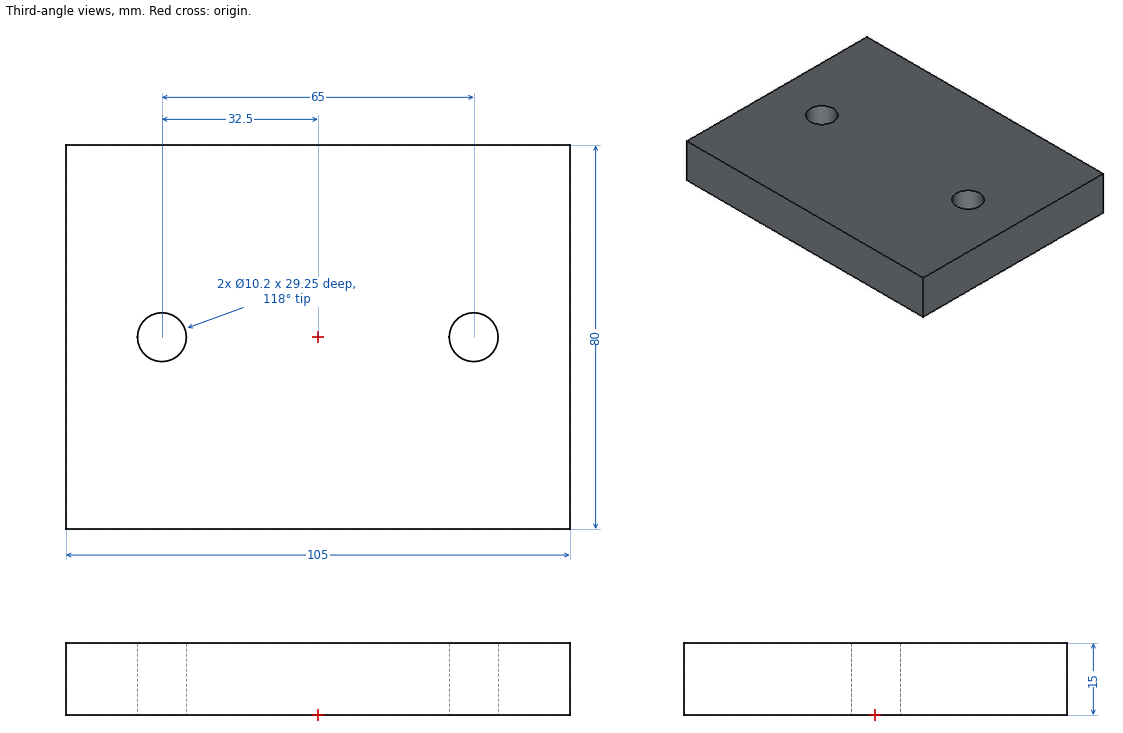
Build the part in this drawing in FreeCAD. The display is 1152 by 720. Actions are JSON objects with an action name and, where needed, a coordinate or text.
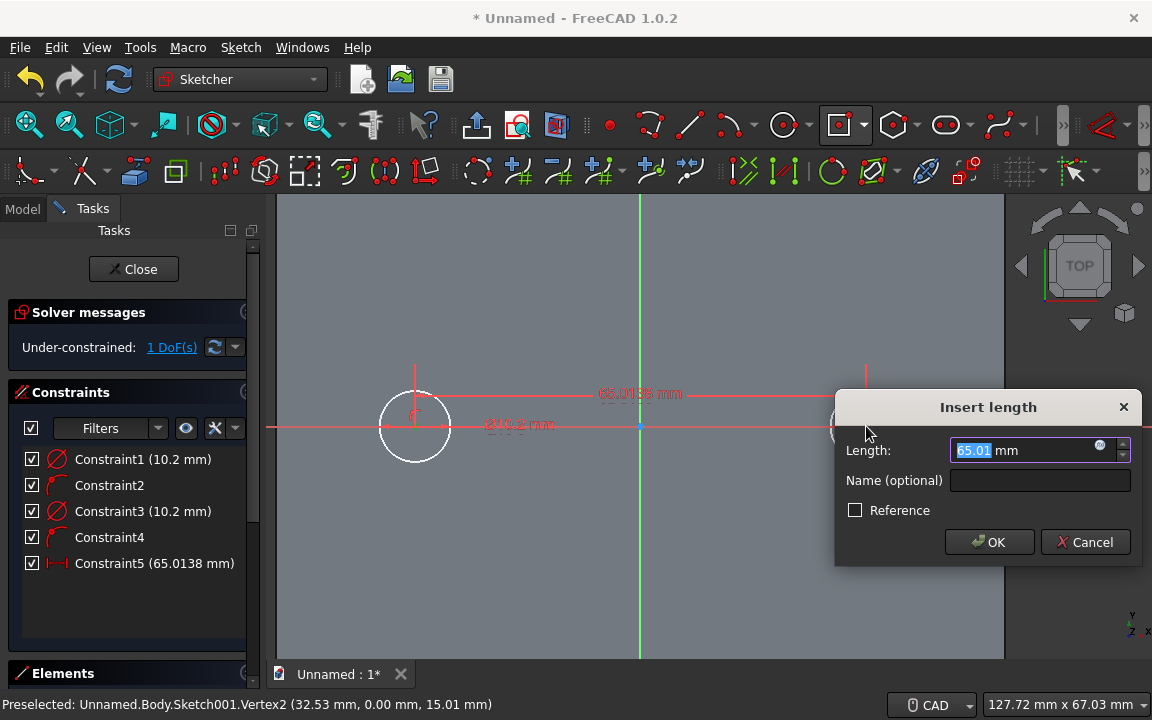
{"action": "type", "text": "65"}
{"action": "key", "text": "Return"}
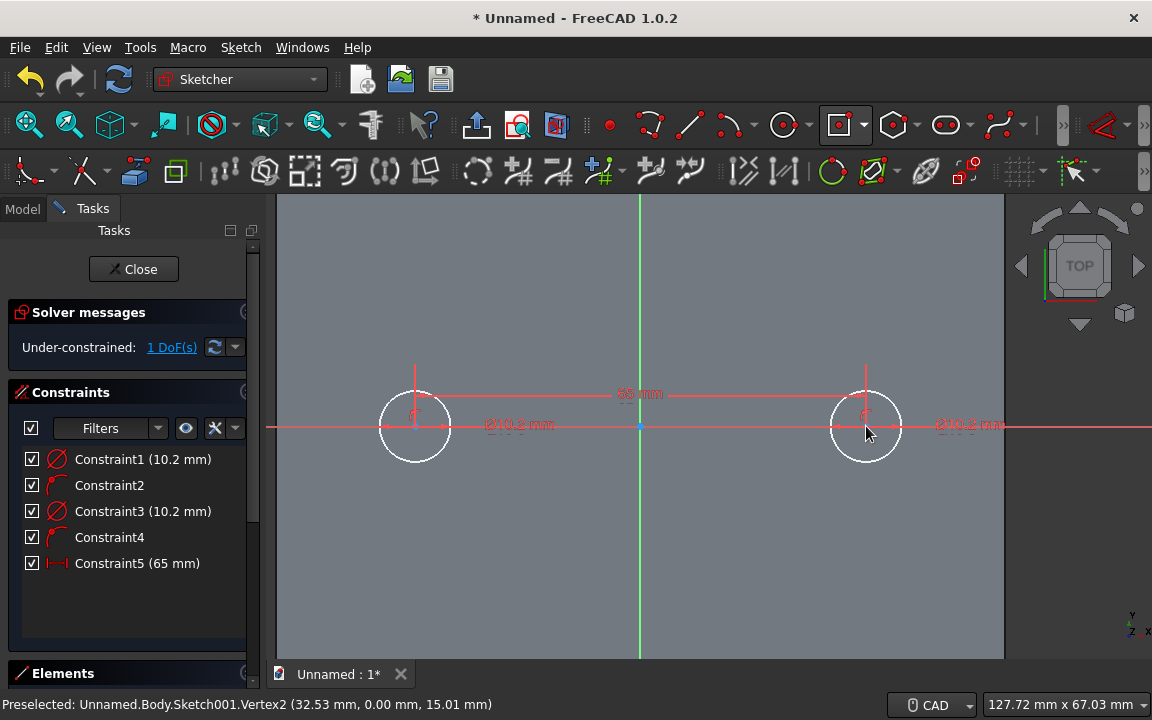
{"action": "left_click", "coordinate": [415, 426]}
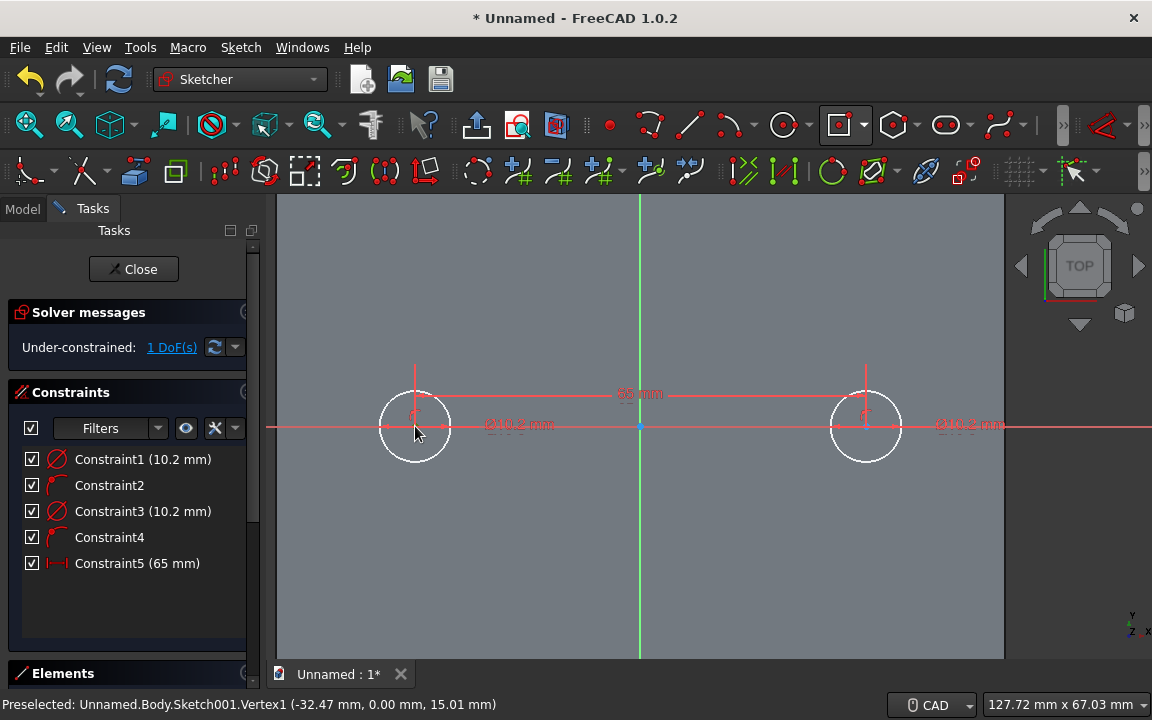
{"action": "left_click", "coordinate": [1130, 126]}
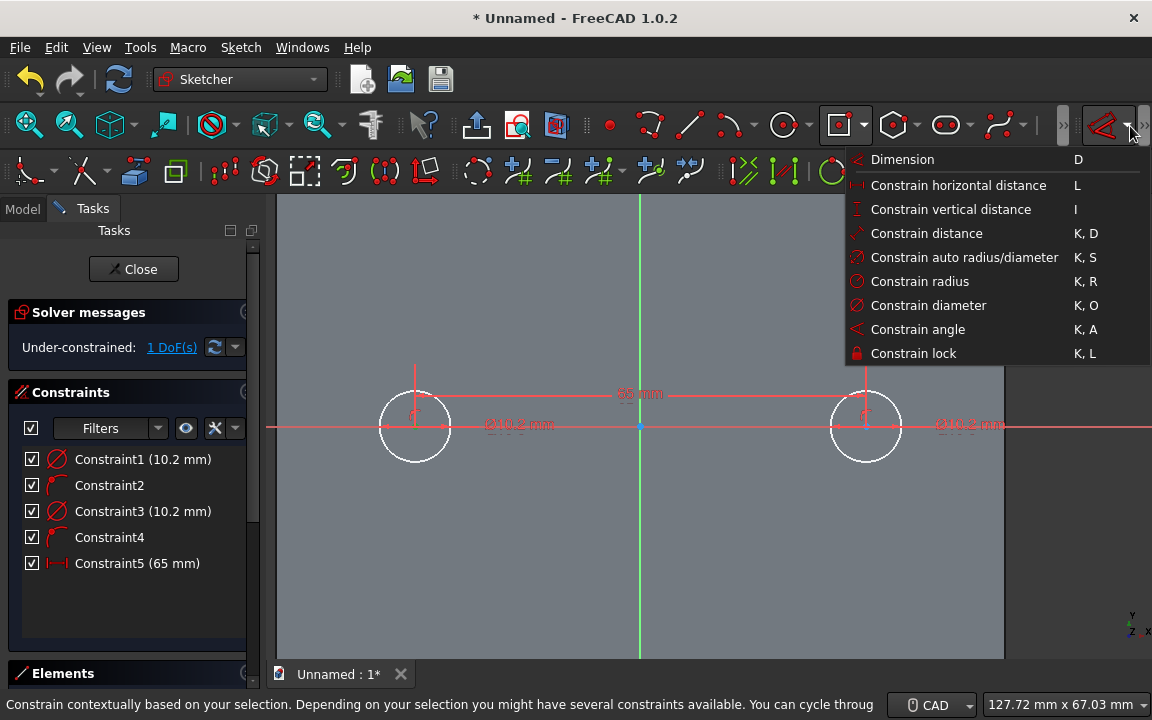
{"action": "left_click", "coordinate": [998, 185]}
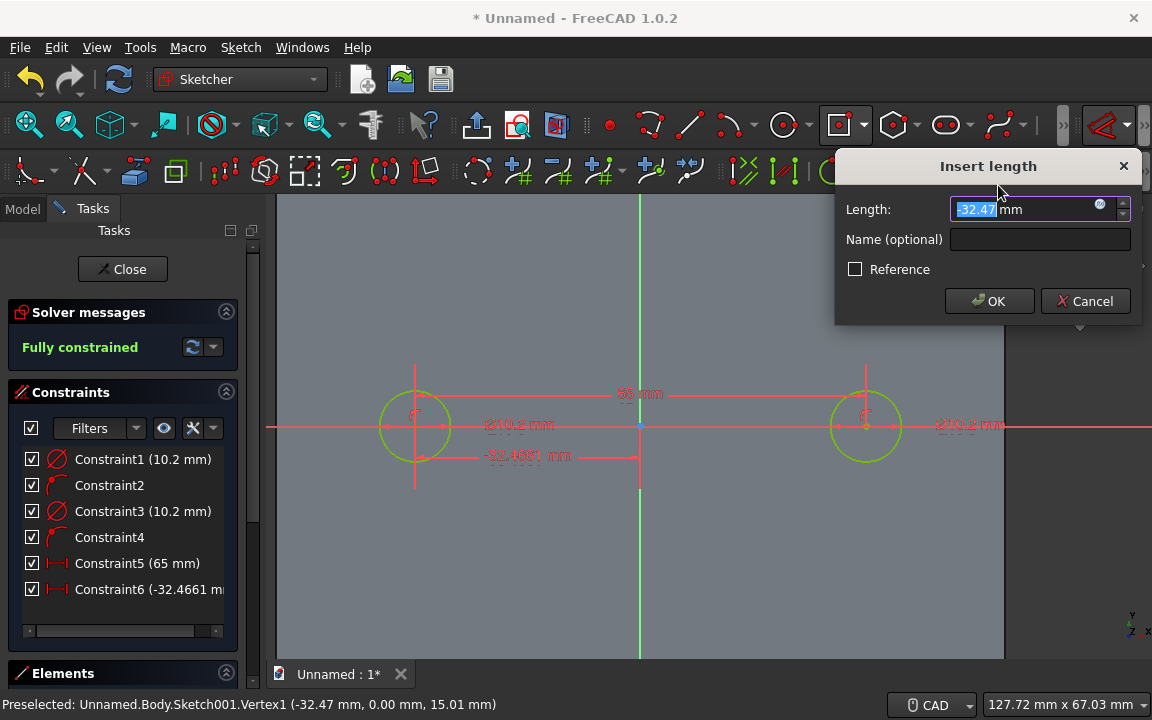
{"action": "type", "text": "-32.5"}
{"action": "key", "text": "Return"}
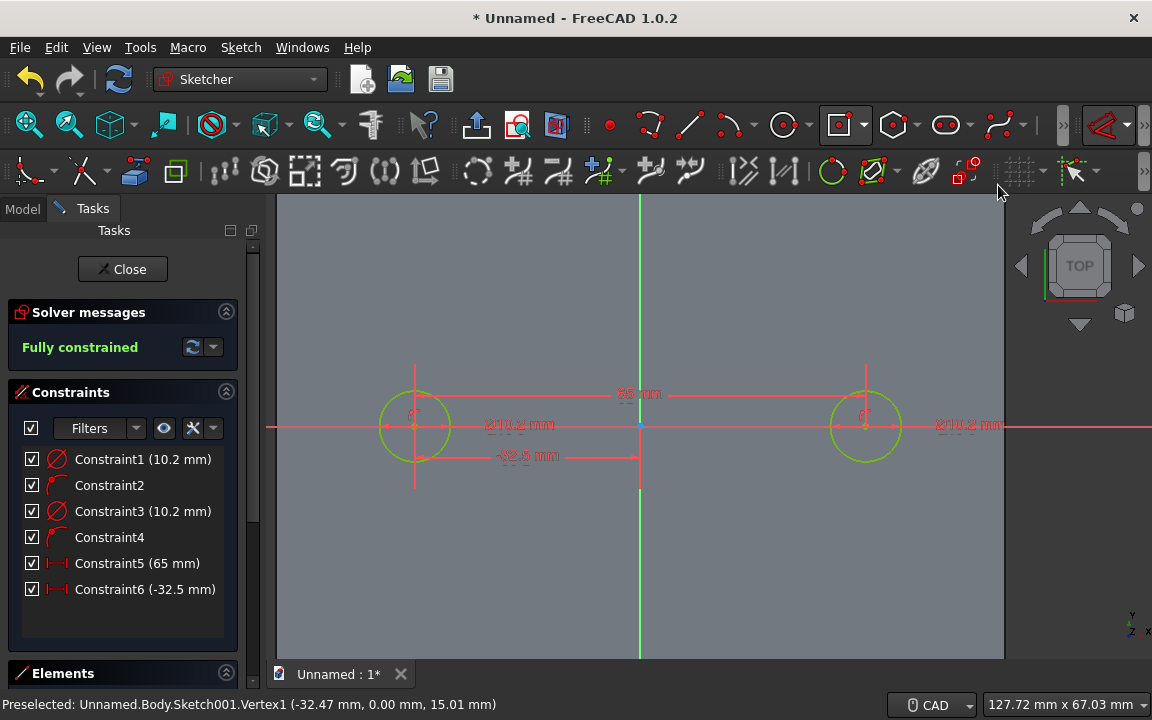
{"action": "left_click", "coordinate": [123, 269]}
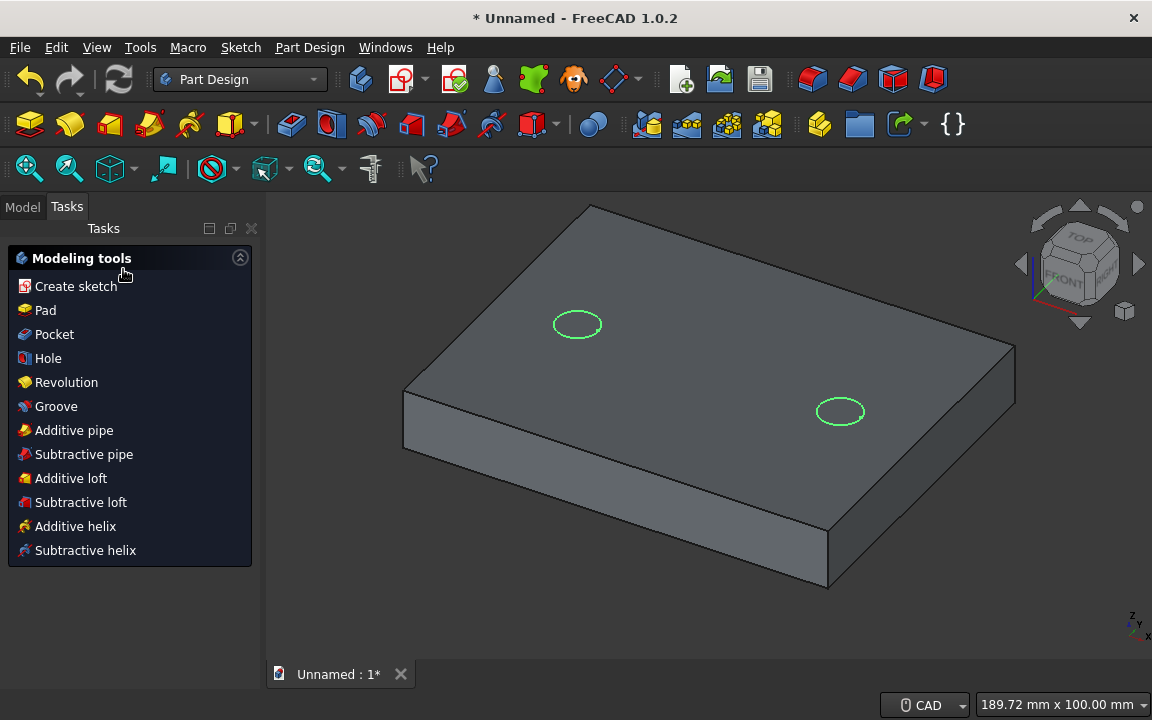
{"action": "left_click", "coordinate": [332, 124]}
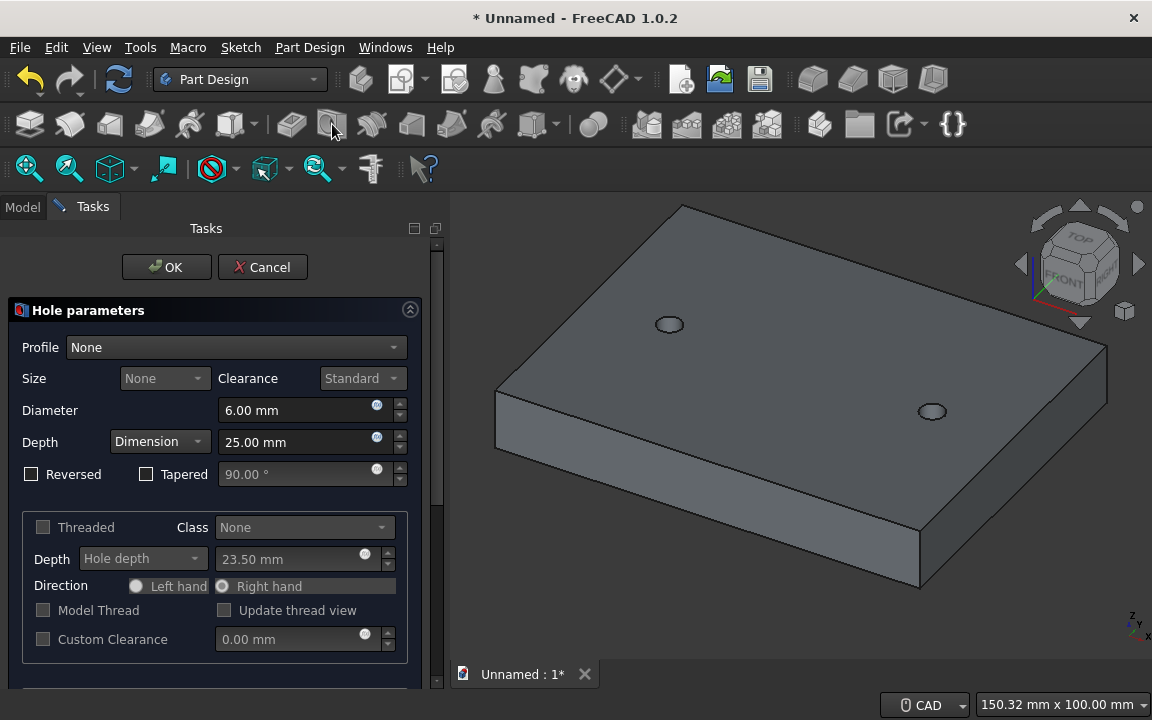
{"action": "triple_click", "coordinate": [305, 410]}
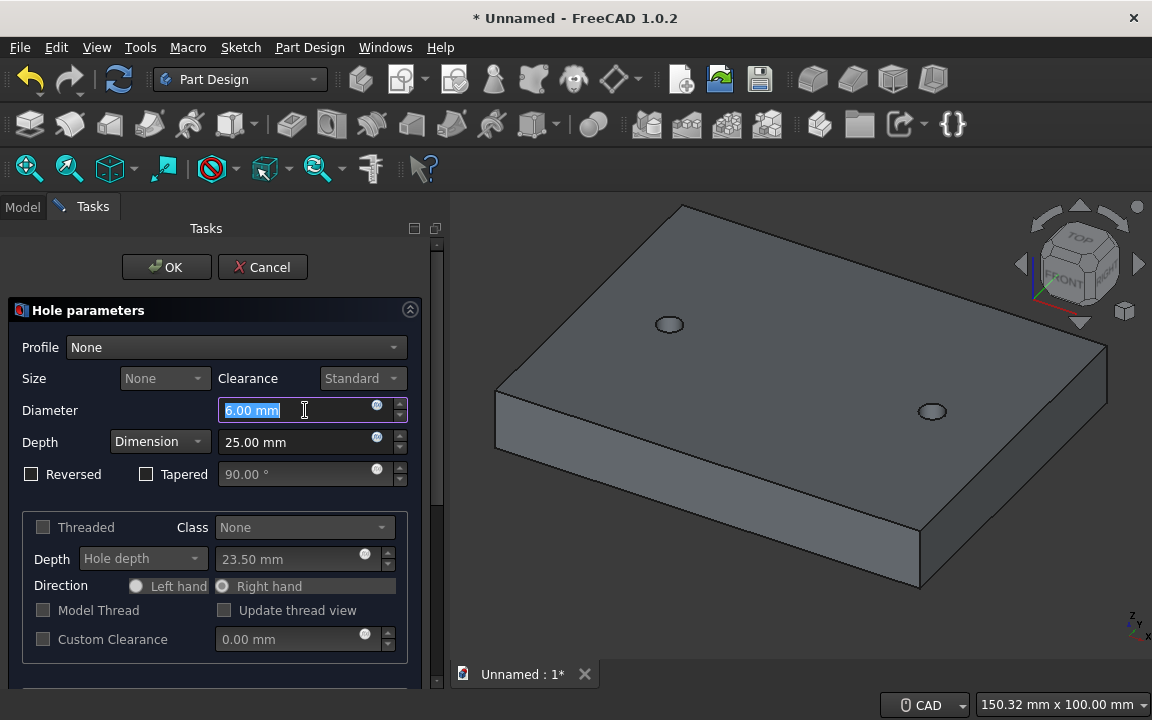
{"action": "type", "text": "10.2"}
{"action": "key", "text": "Tab"}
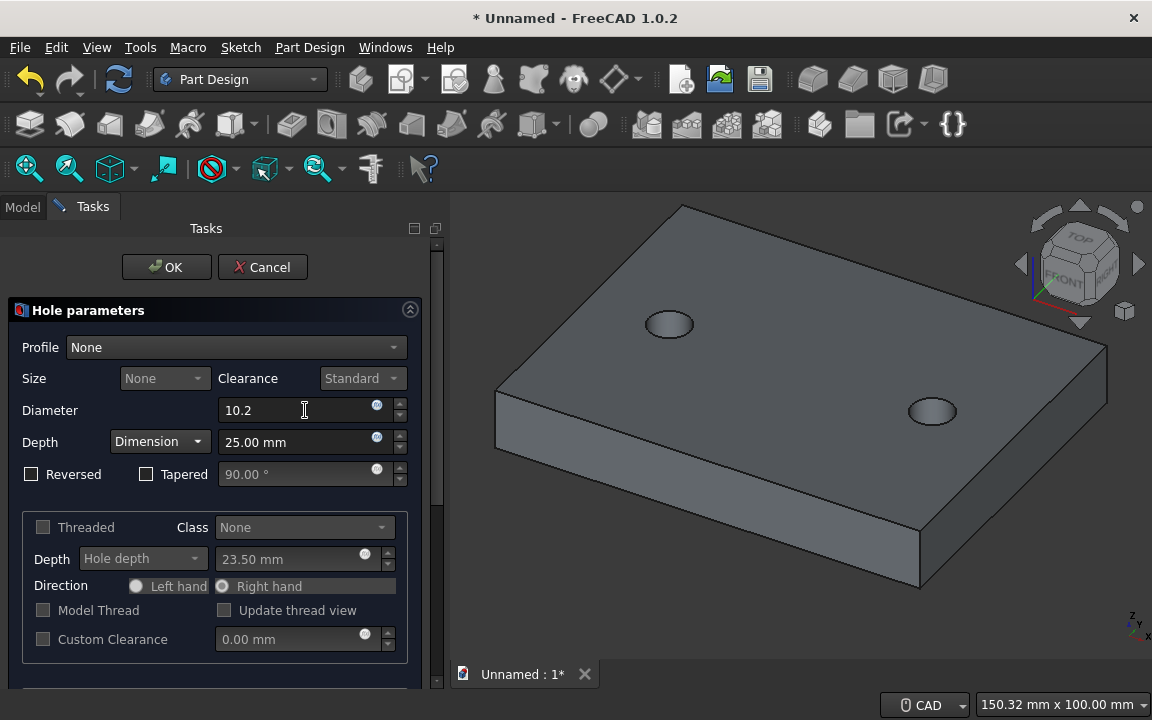
{"action": "triple_click", "coordinate": [305, 442]}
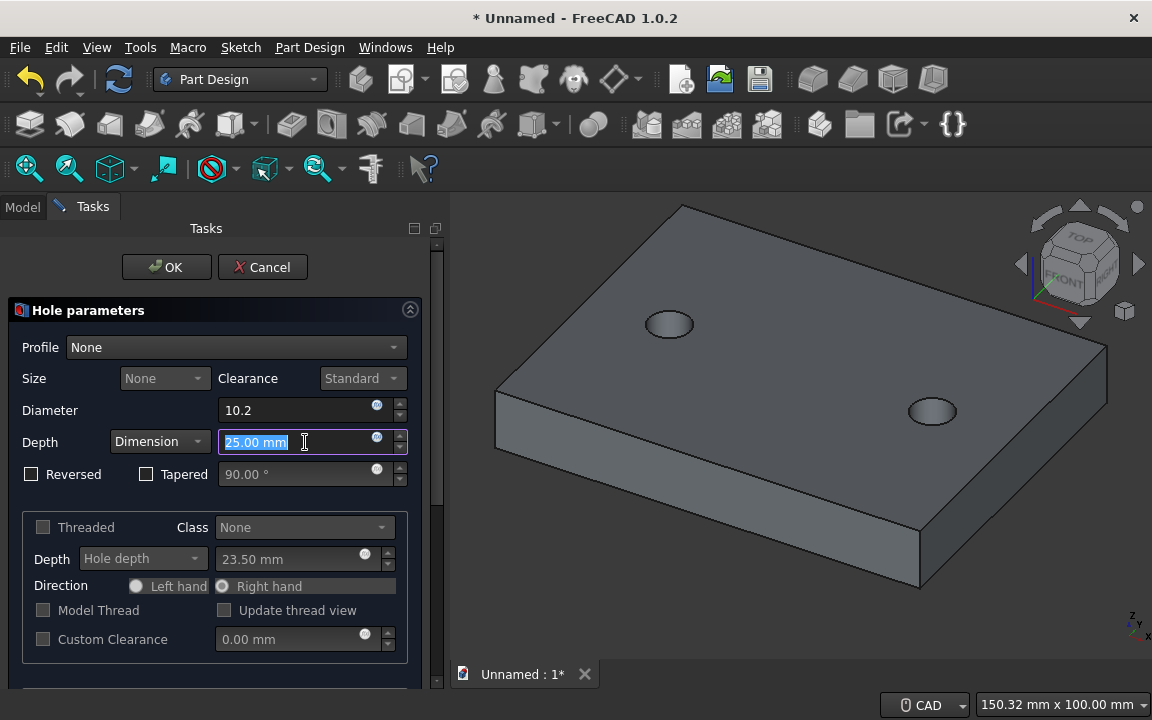
{"action": "type", "text": "29.25"}
{"action": "key", "text": "Tab"}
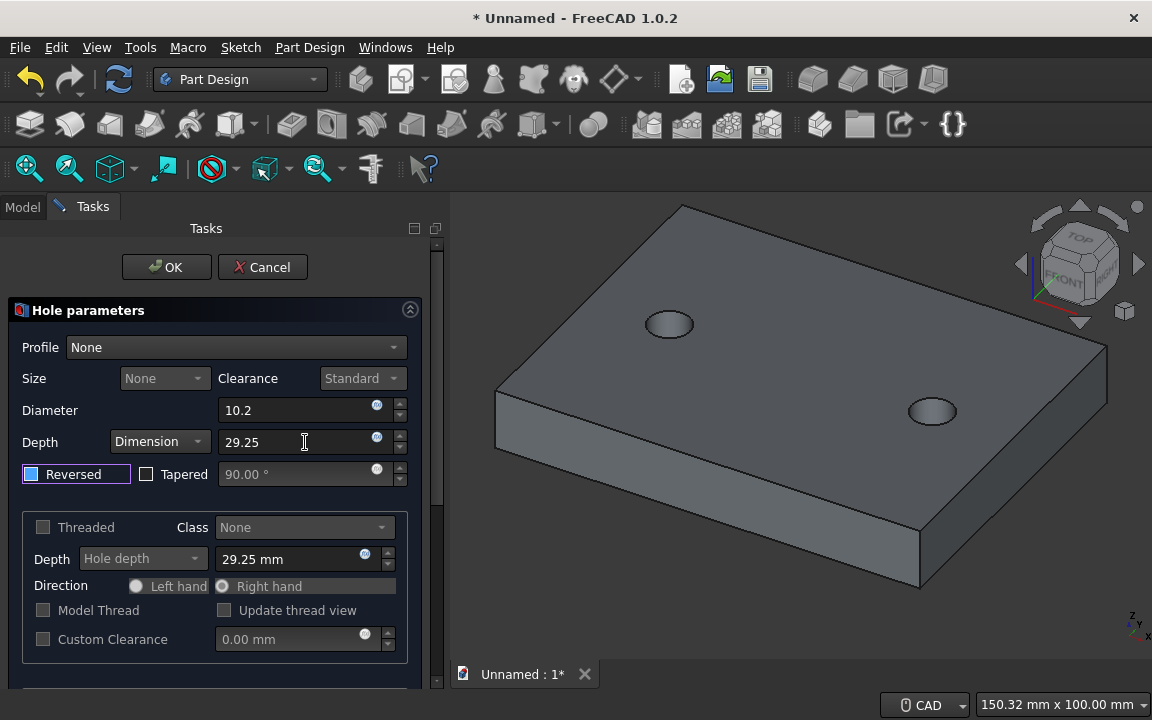
{"action": "left_click", "coordinate": [167, 267]}